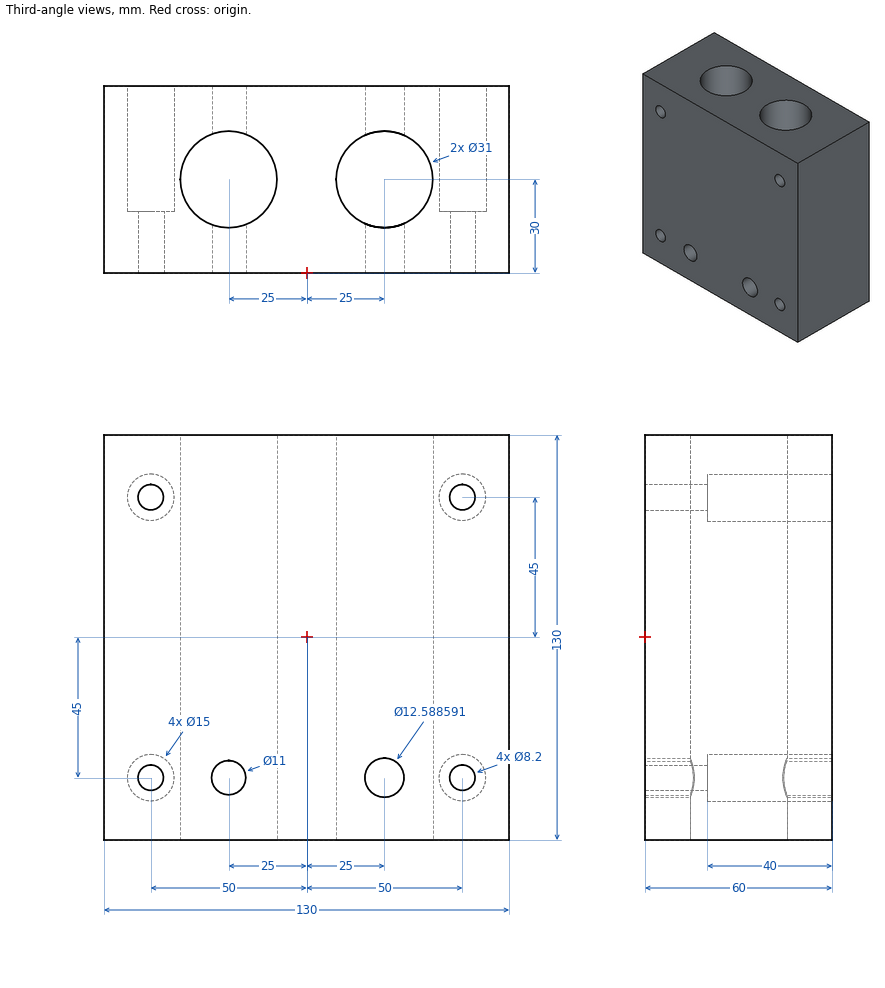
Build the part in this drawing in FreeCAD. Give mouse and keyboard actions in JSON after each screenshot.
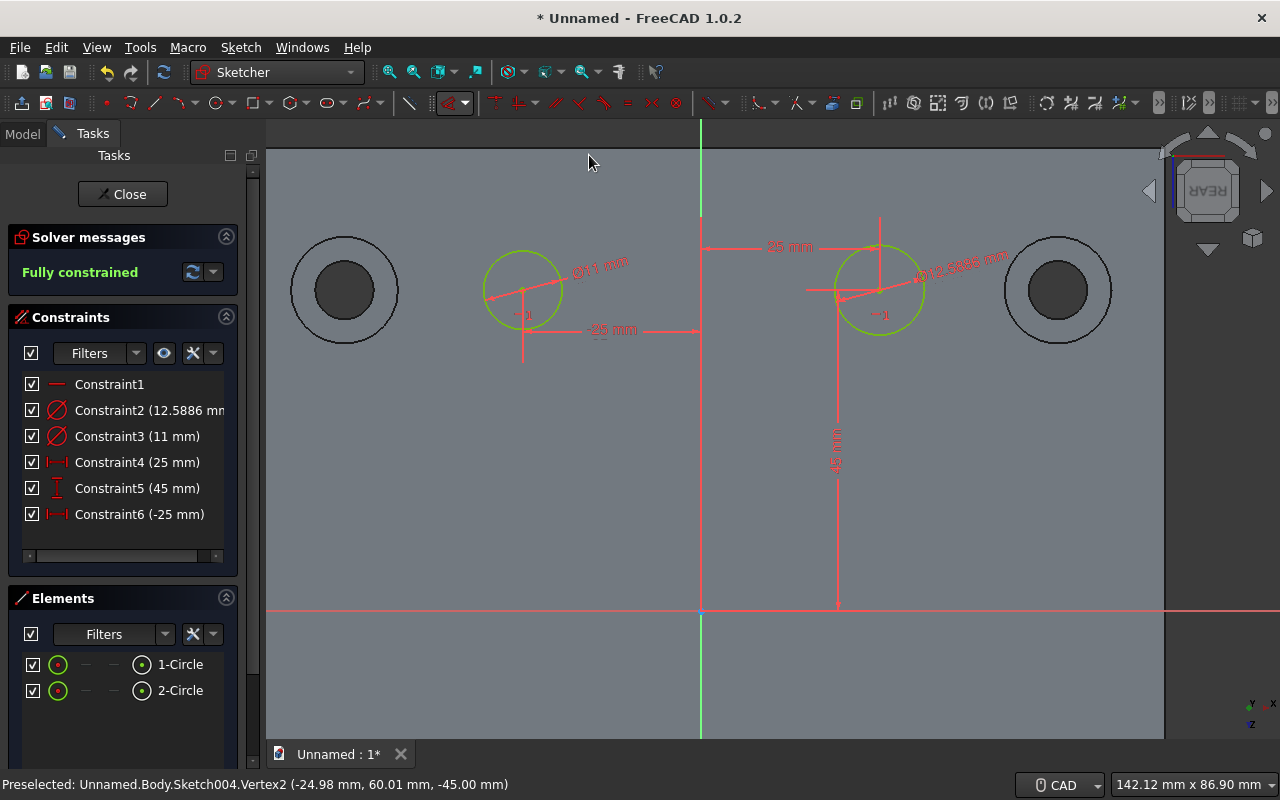
{"action": "left_click", "coordinate": [123, 194]}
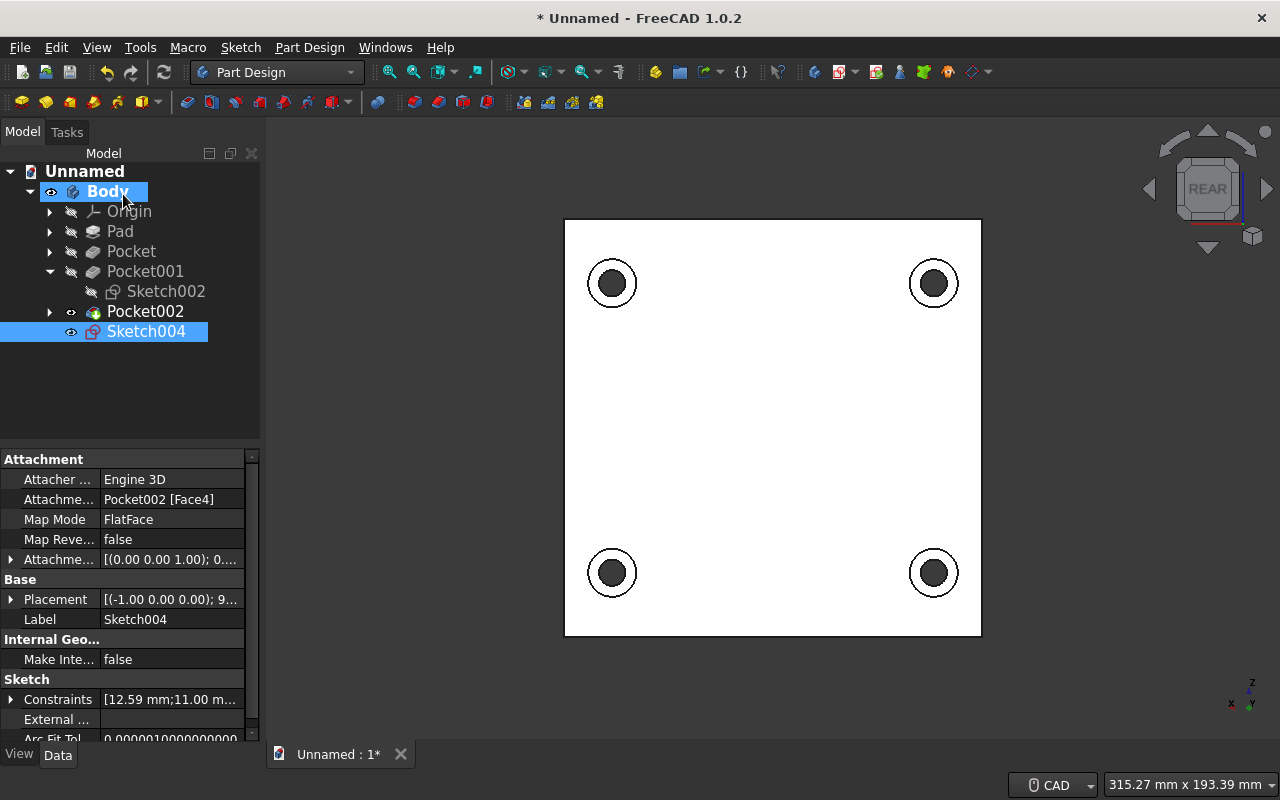
{"action": "left_click", "coordinate": [188, 102]}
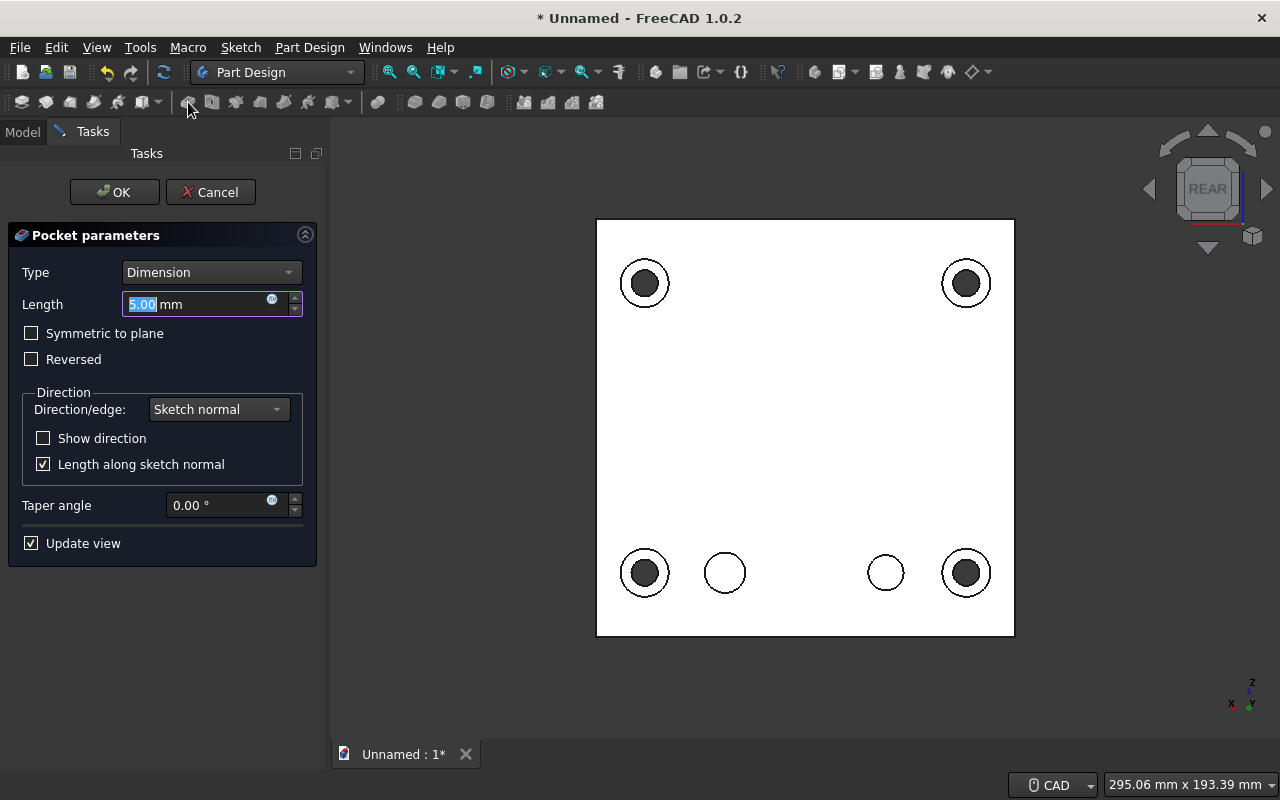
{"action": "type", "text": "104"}
{"action": "key", "text": "Tab"}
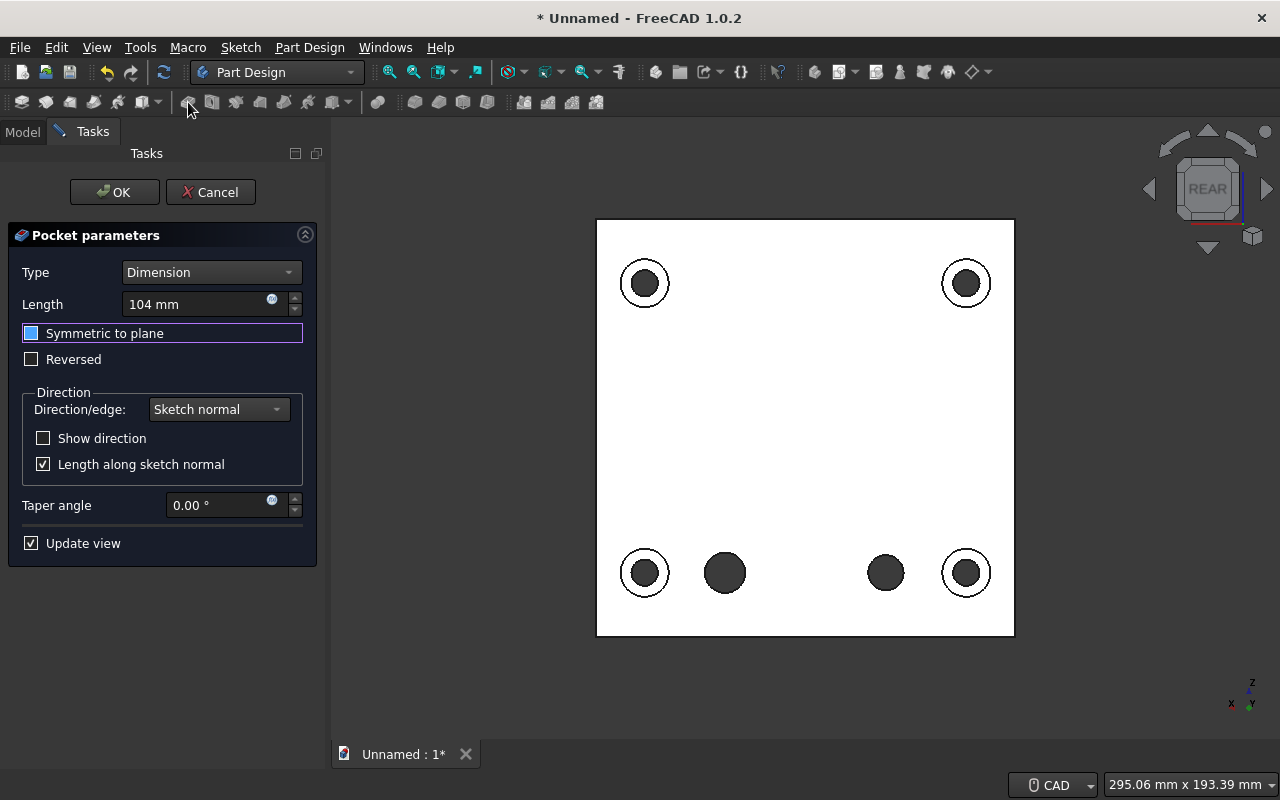
{"action": "left_click", "coordinate": [115, 192]}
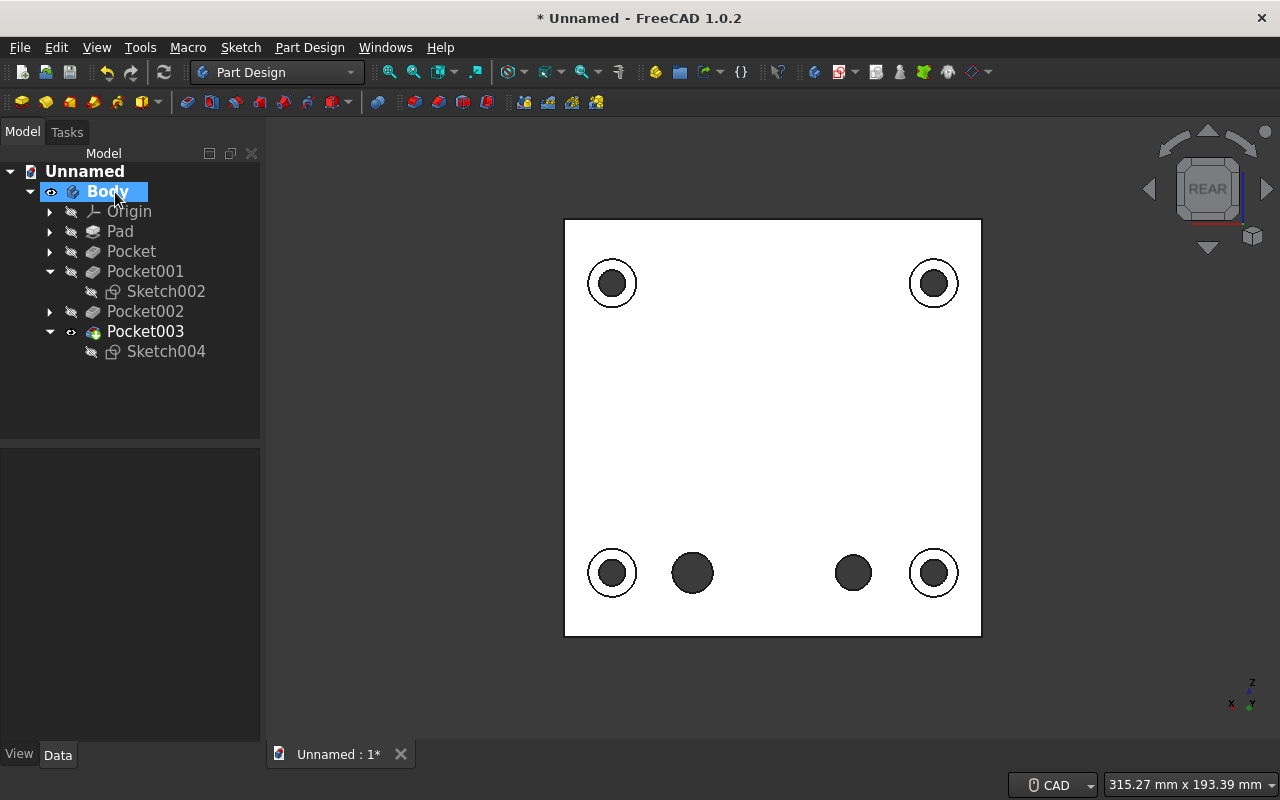
{"action": "key", "text": "0"}